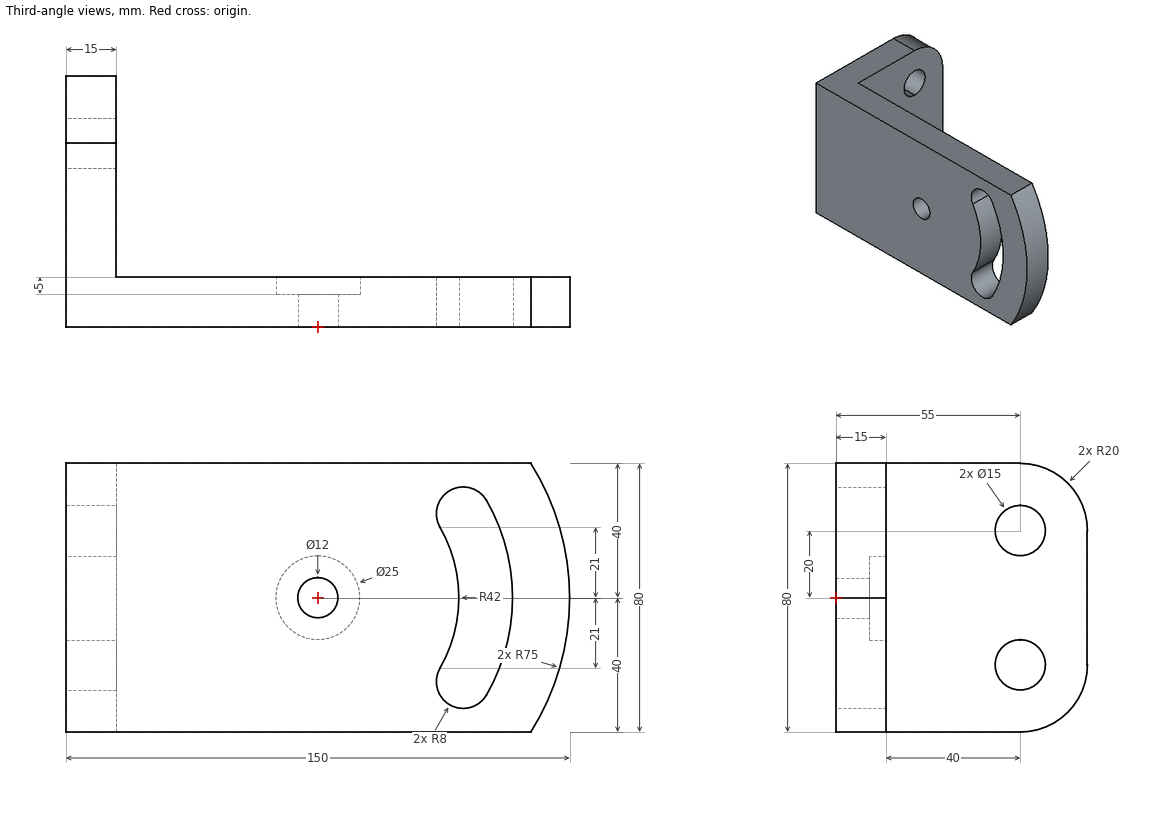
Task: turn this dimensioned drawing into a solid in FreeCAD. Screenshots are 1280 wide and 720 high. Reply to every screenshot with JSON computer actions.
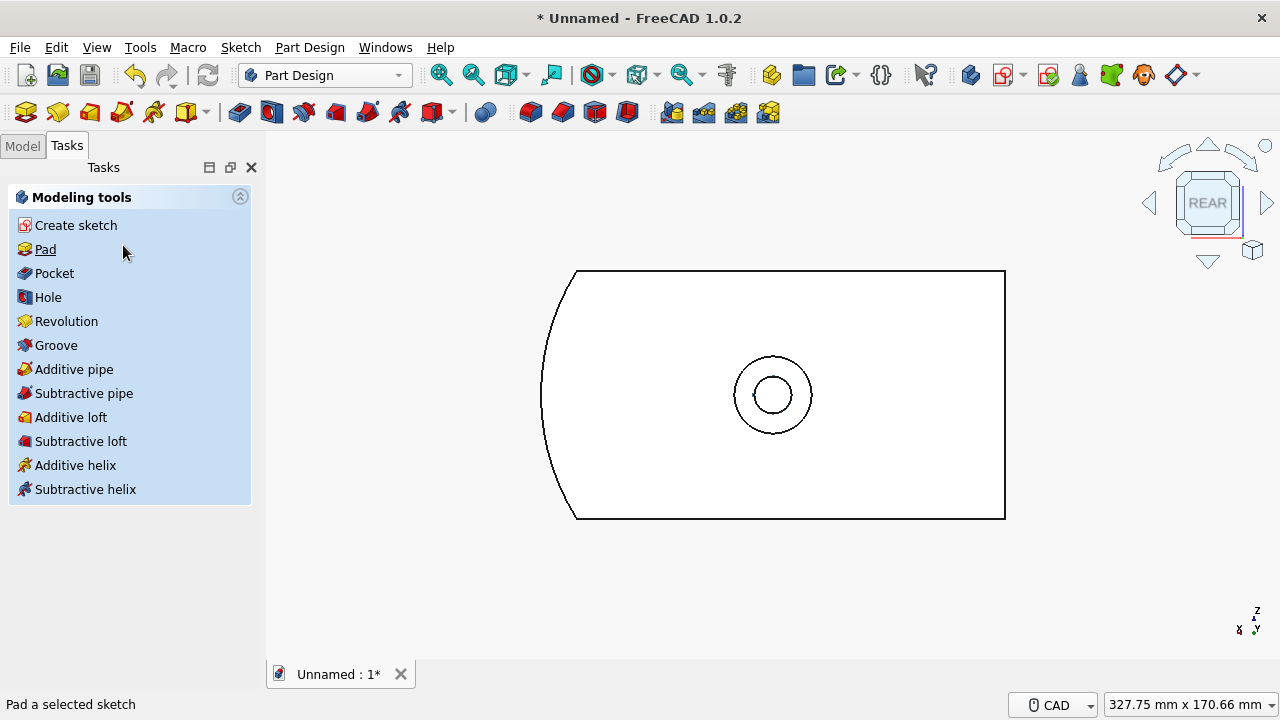
{"action": "left_click", "coordinate": [240, 112]}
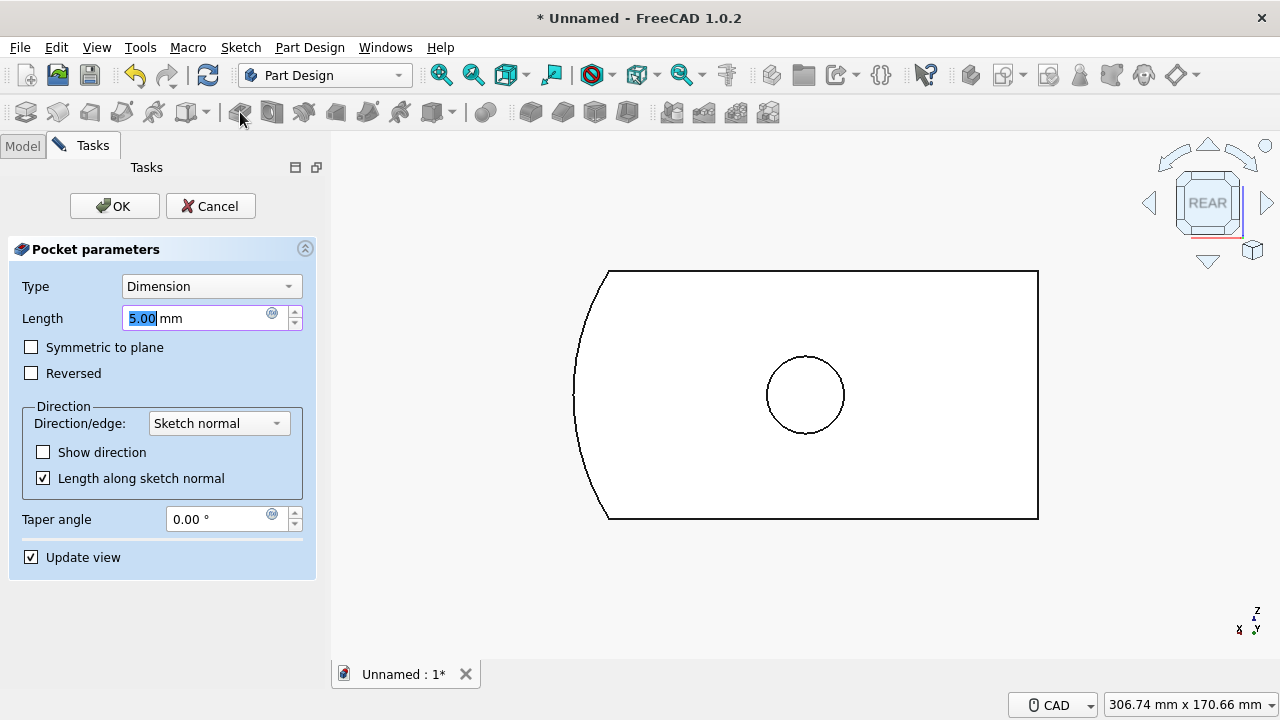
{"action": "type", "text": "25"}
{"action": "key", "text": "Tab"}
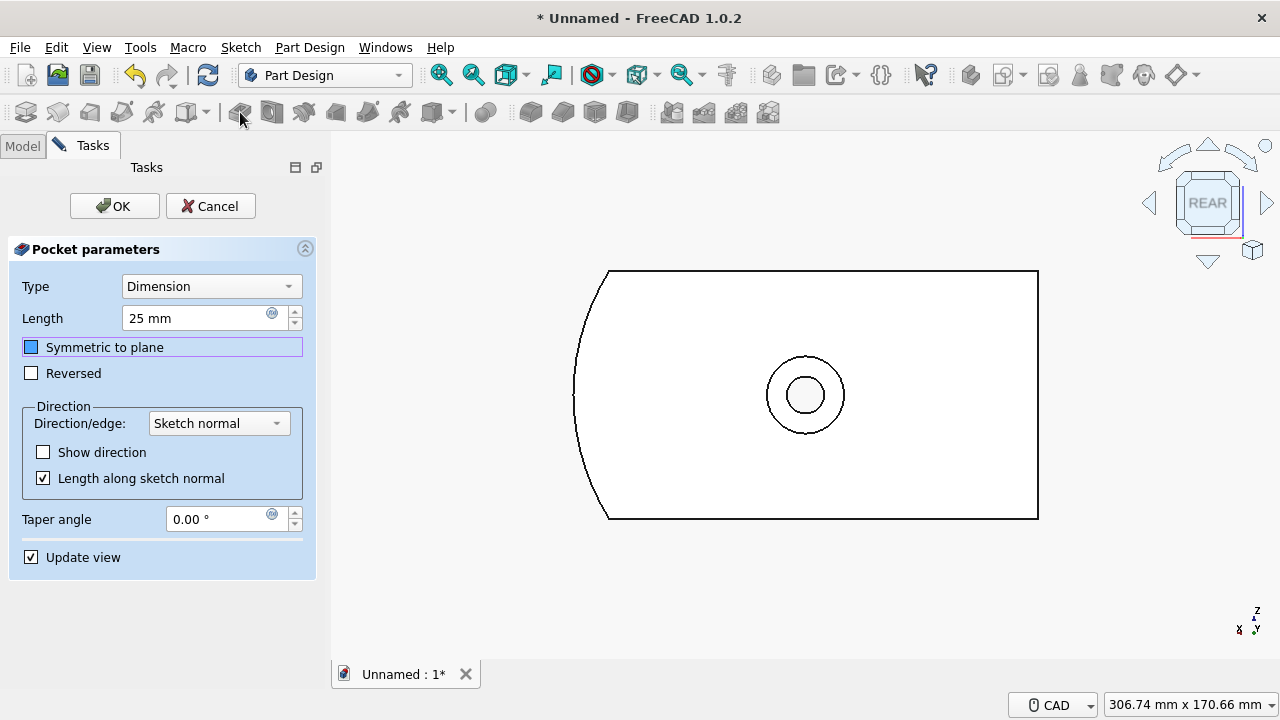
{"action": "left_click", "coordinate": [115, 206]}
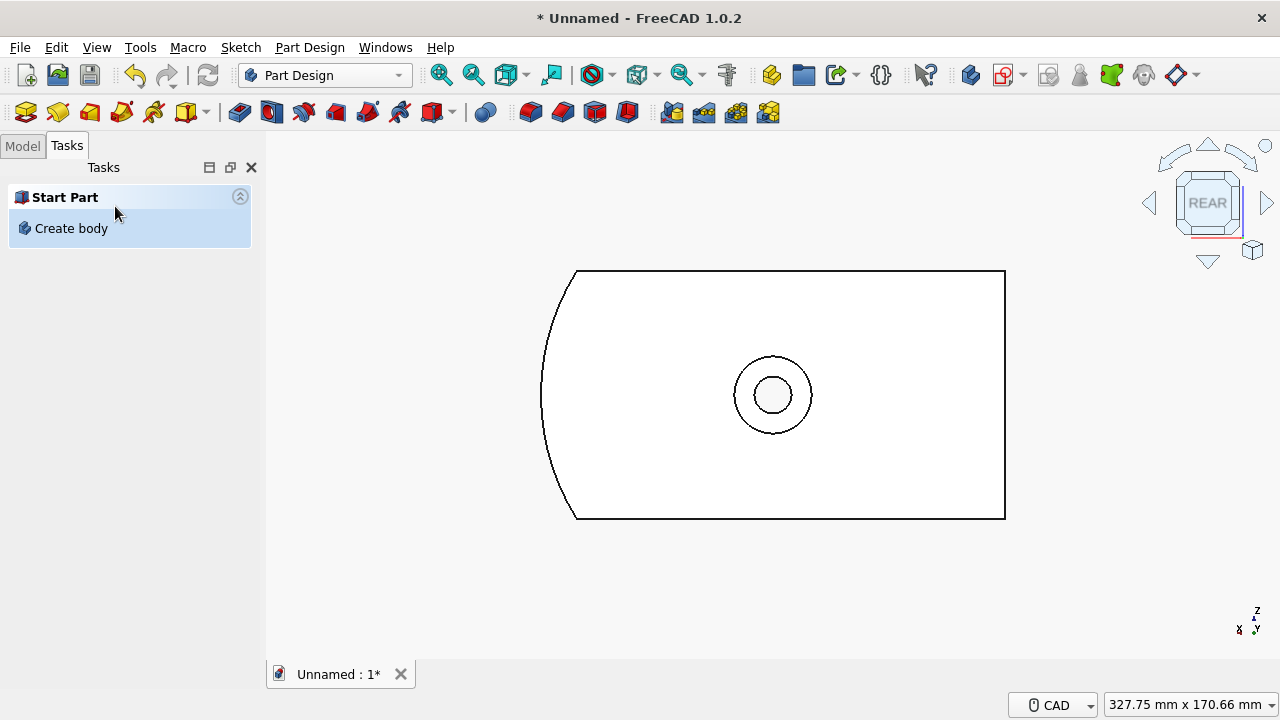
{"action": "left_click", "coordinate": [762, 416]}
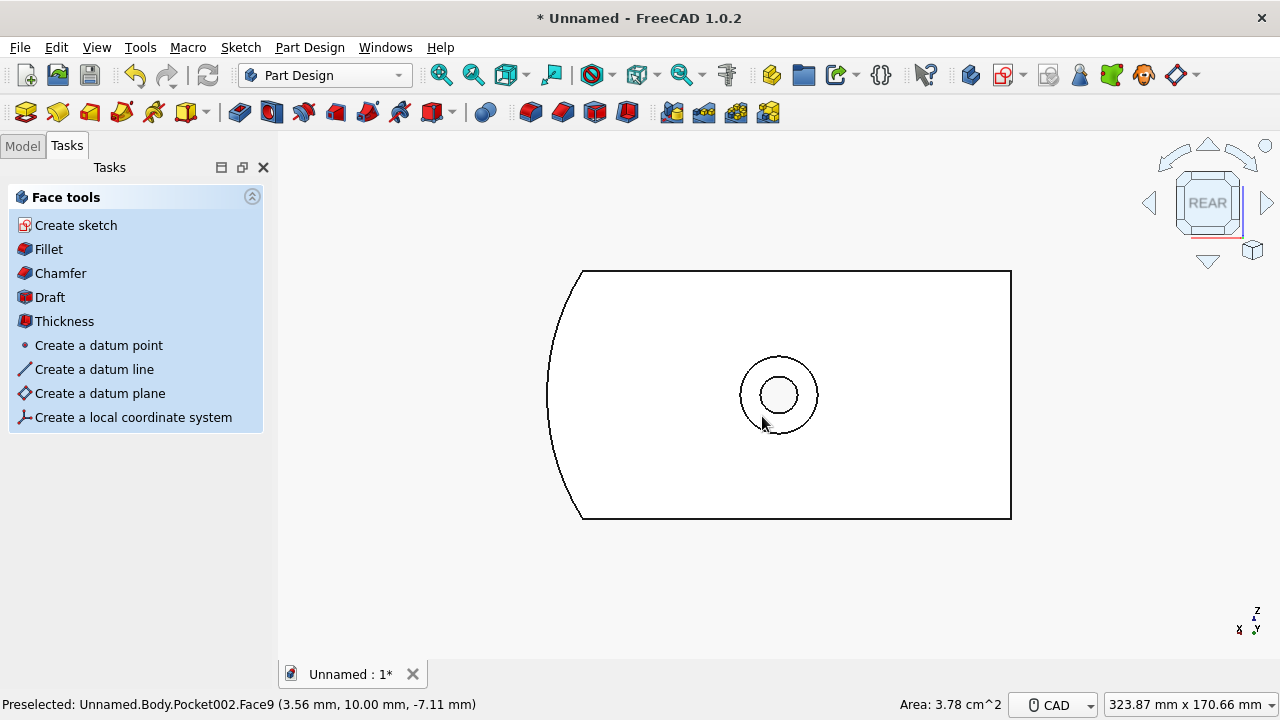
{"action": "left_click", "coordinate": [1004, 76]}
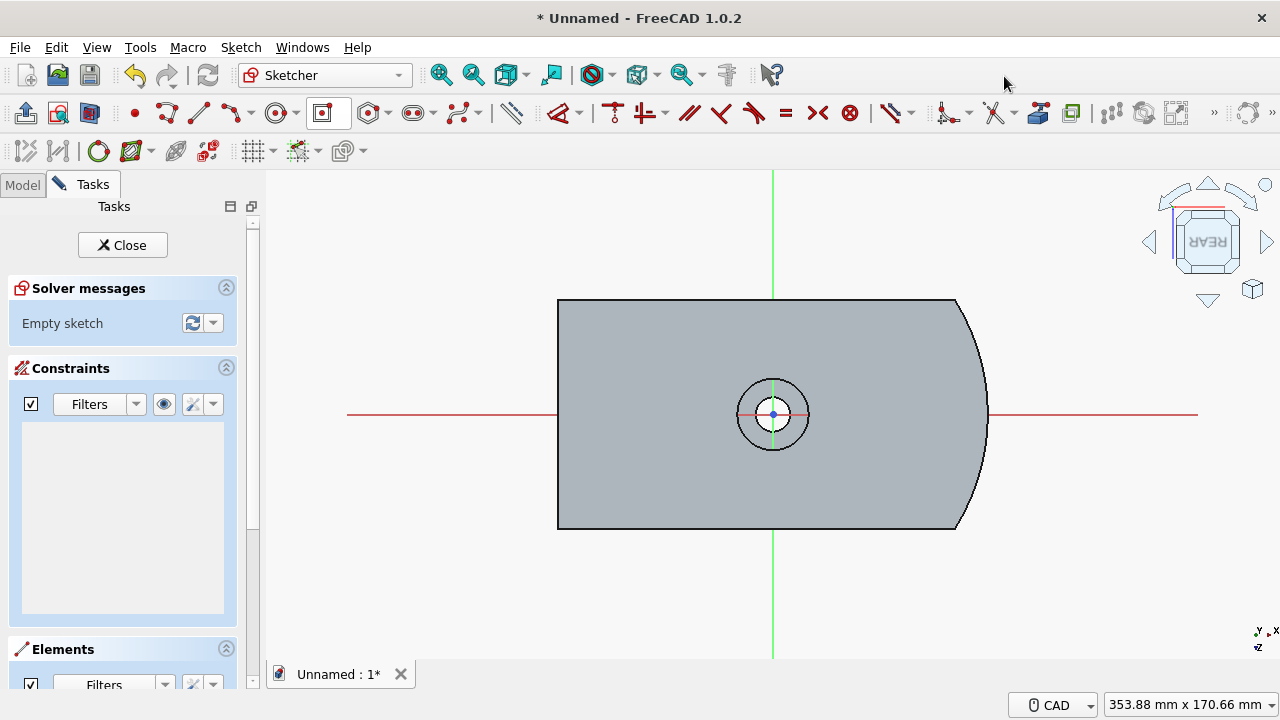
{"action": "left_click", "coordinate": [90, 114]}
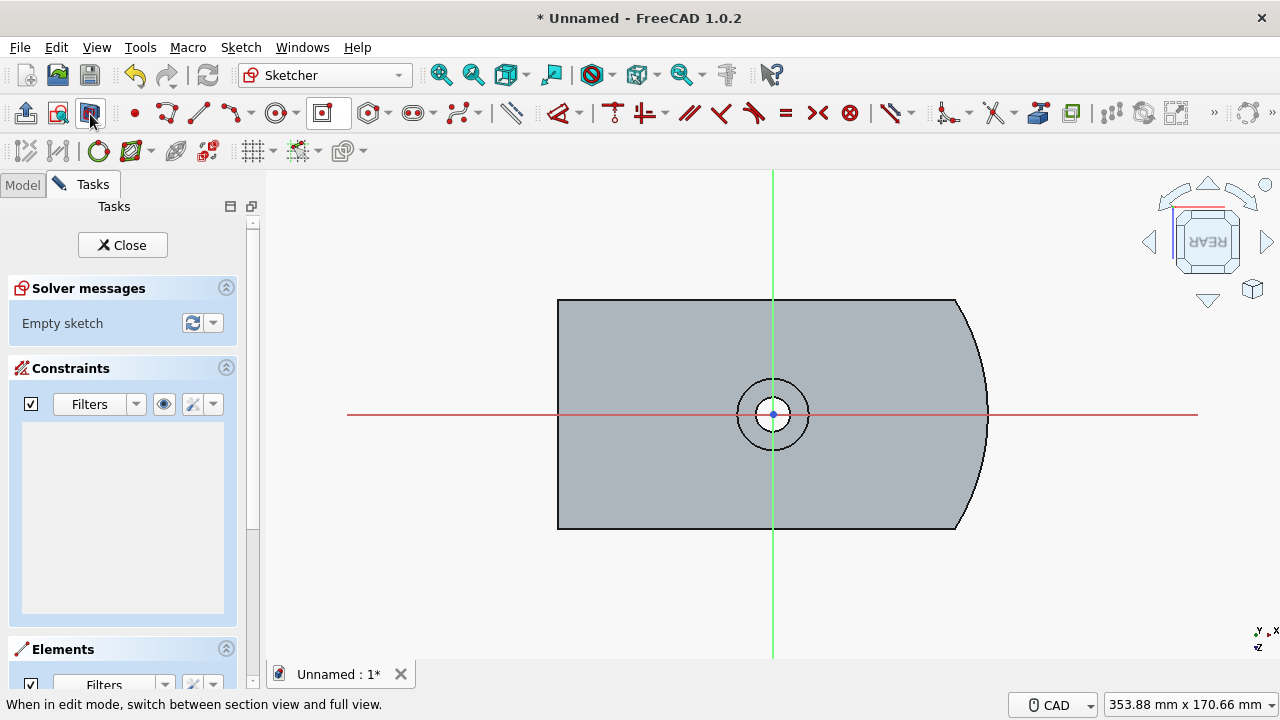
{"action": "scroll", "coordinate": [1040, 414], "scroll_direction": "up", "scroll_amount": 3}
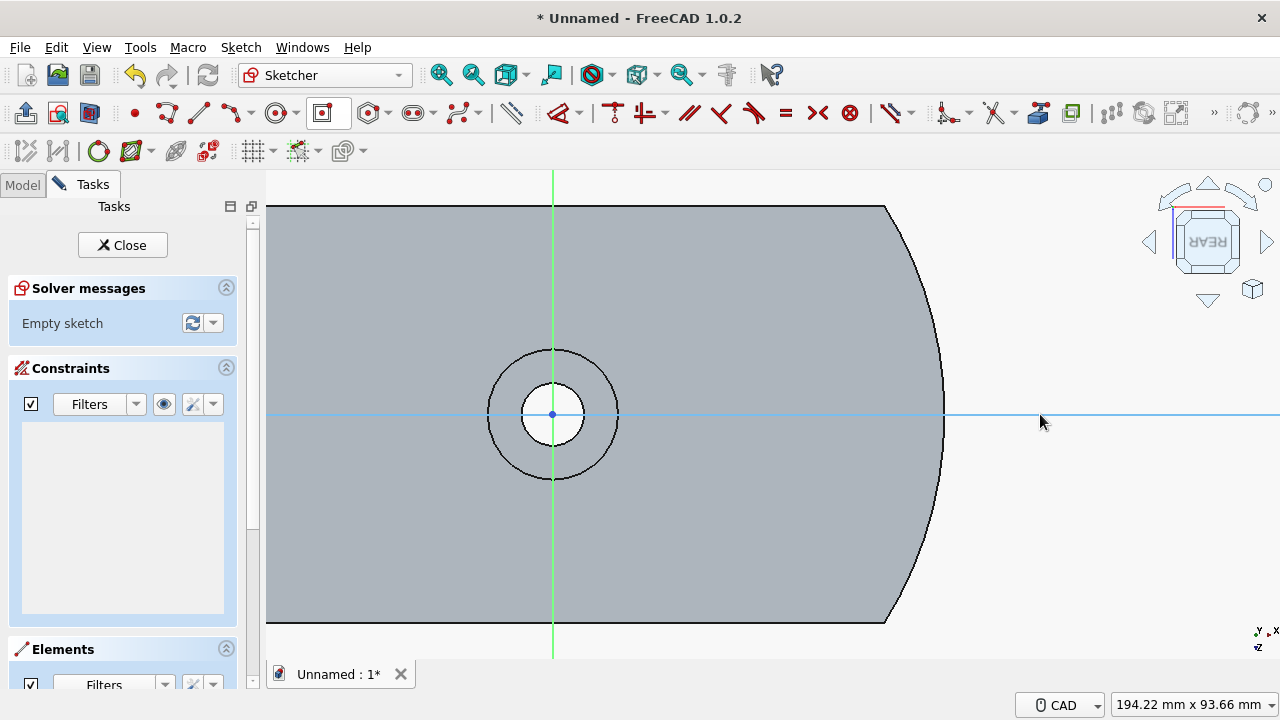
{"action": "key", "text": "g 3 a"}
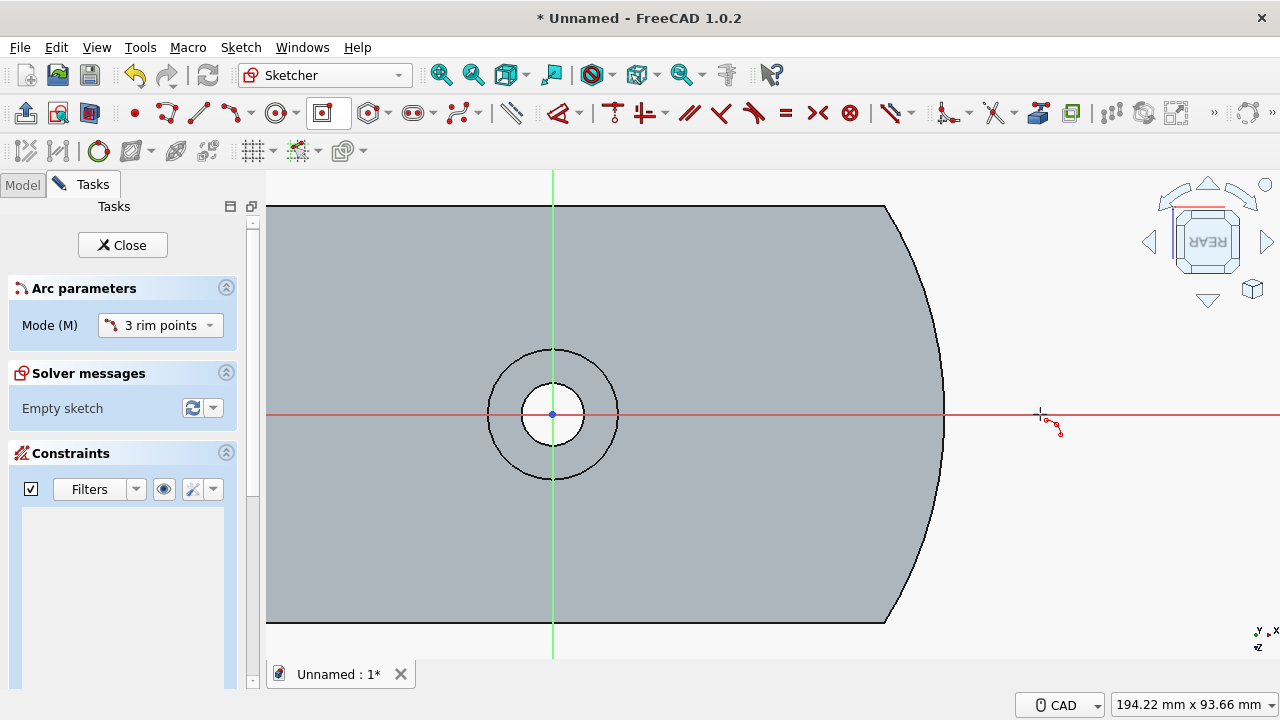
{"action": "left_click", "coordinate": [743, 305]}
{"action": "left_click", "coordinate": [743, 524]}
{"action": "left_click", "coordinate": [771, 437]}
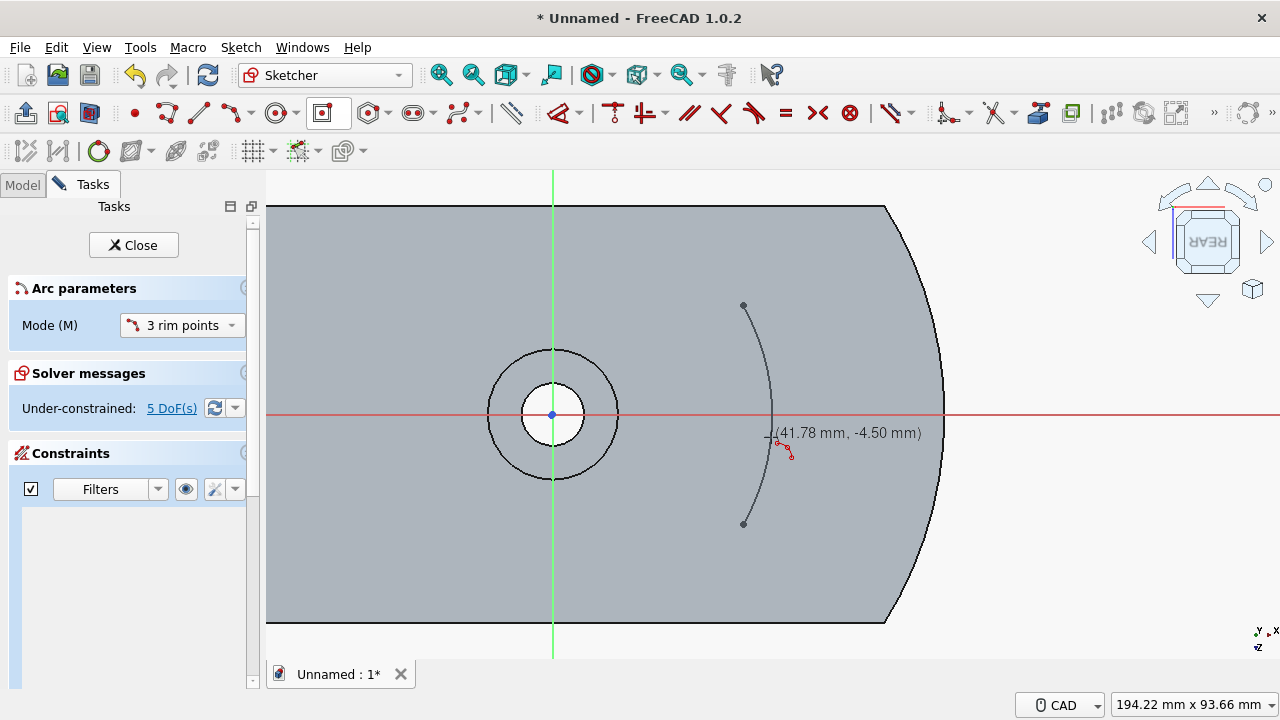
{"action": "left_click", "coordinate": [743, 525]}
{"action": "left_click", "coordinate": [815, 566]}
{"action": "left_click", "coordinate": [758, 581]}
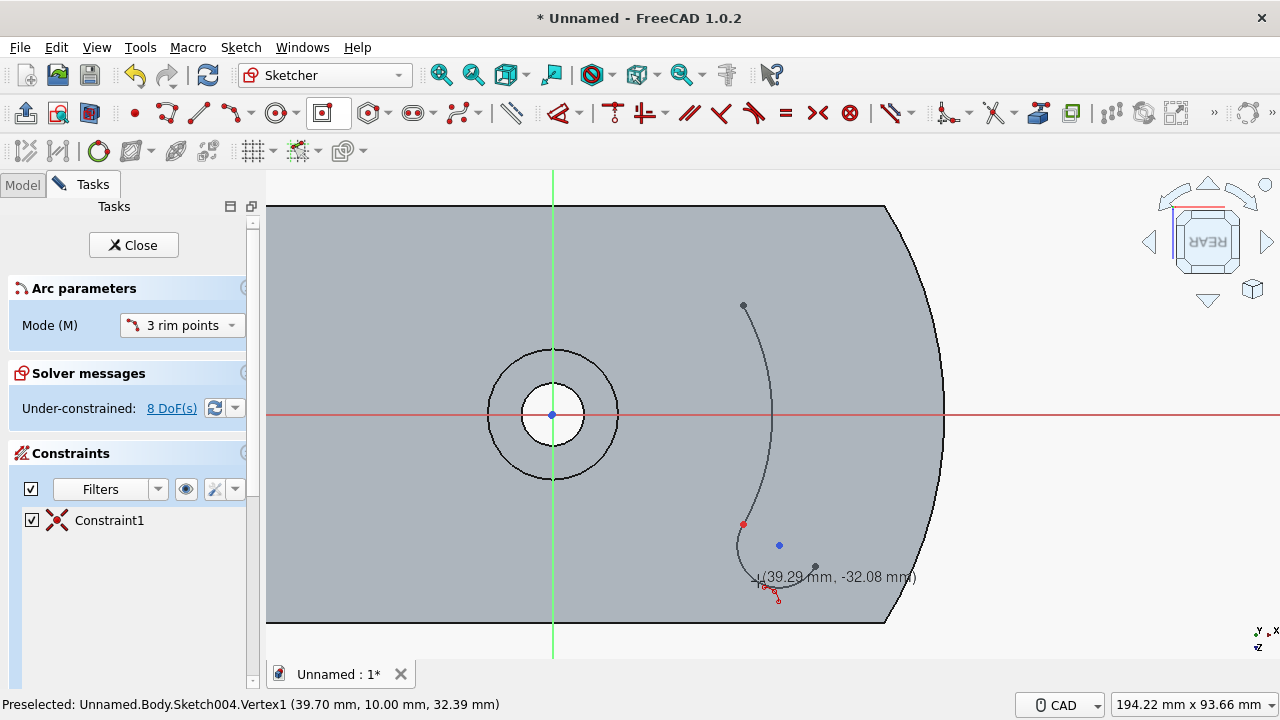
{"action": "left_click", "coordinate": [815, 567]}
{"action": "left_click", "coordinate": [815, 263]}
{"action": "left_click", "coordinate": [854, 446]}